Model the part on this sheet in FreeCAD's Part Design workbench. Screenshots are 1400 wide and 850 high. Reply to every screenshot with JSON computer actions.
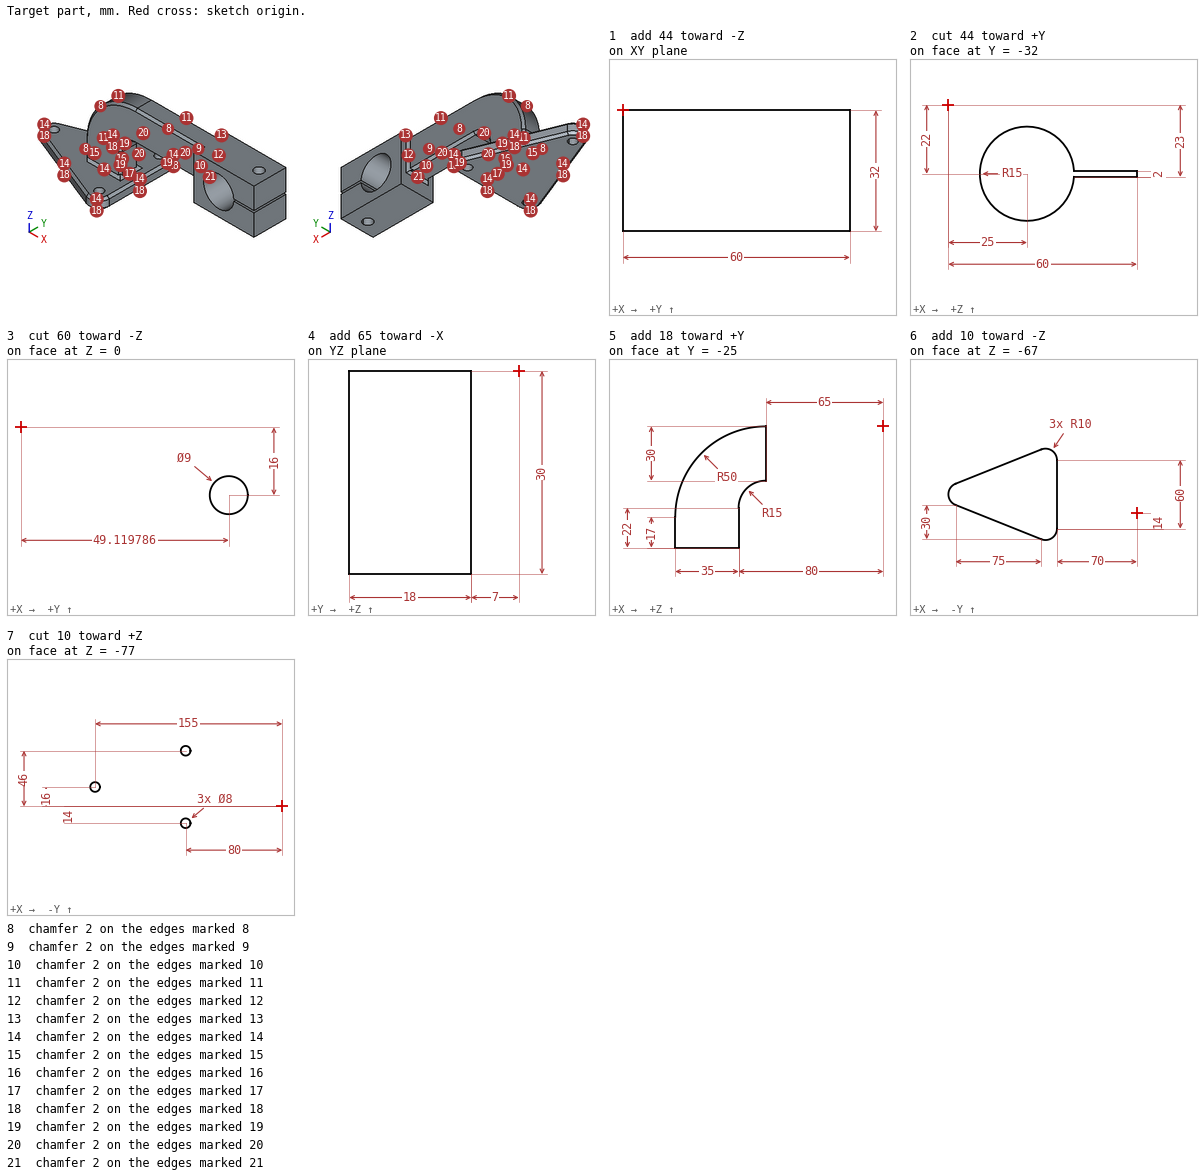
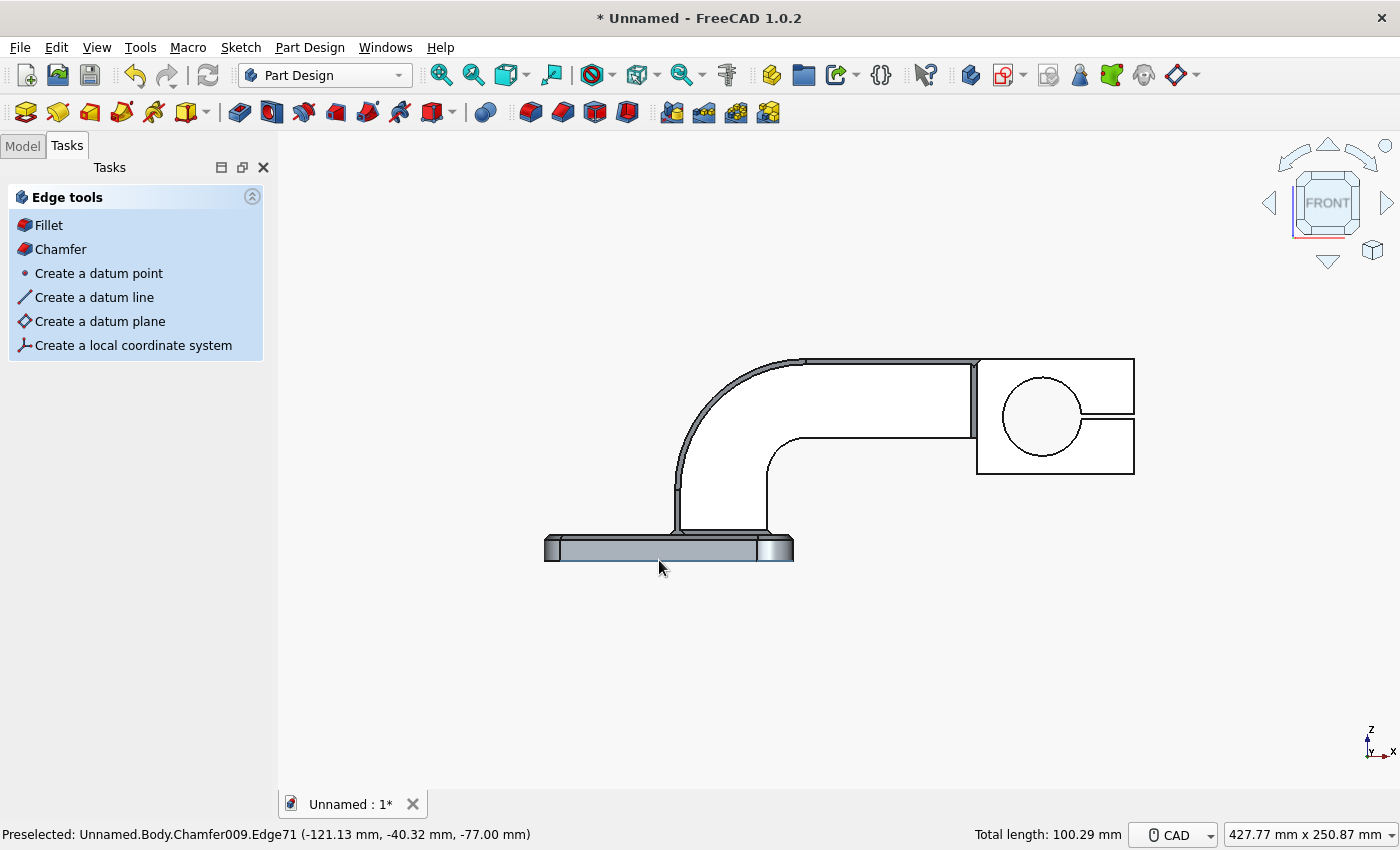
{"action": "left_click", "coordinate": [544, 560], "text": "ctrl"}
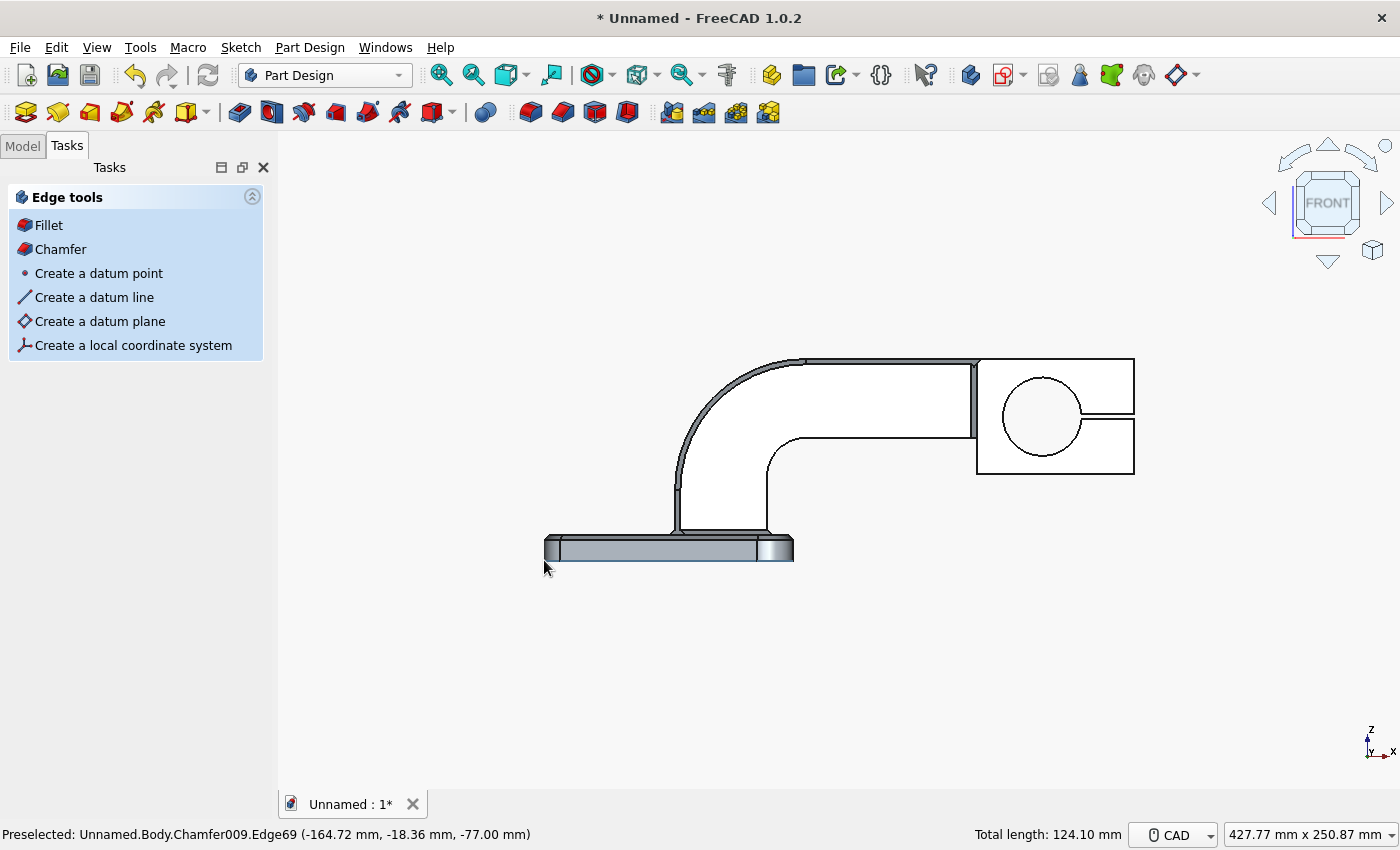
{"action": "key", "text": "3"}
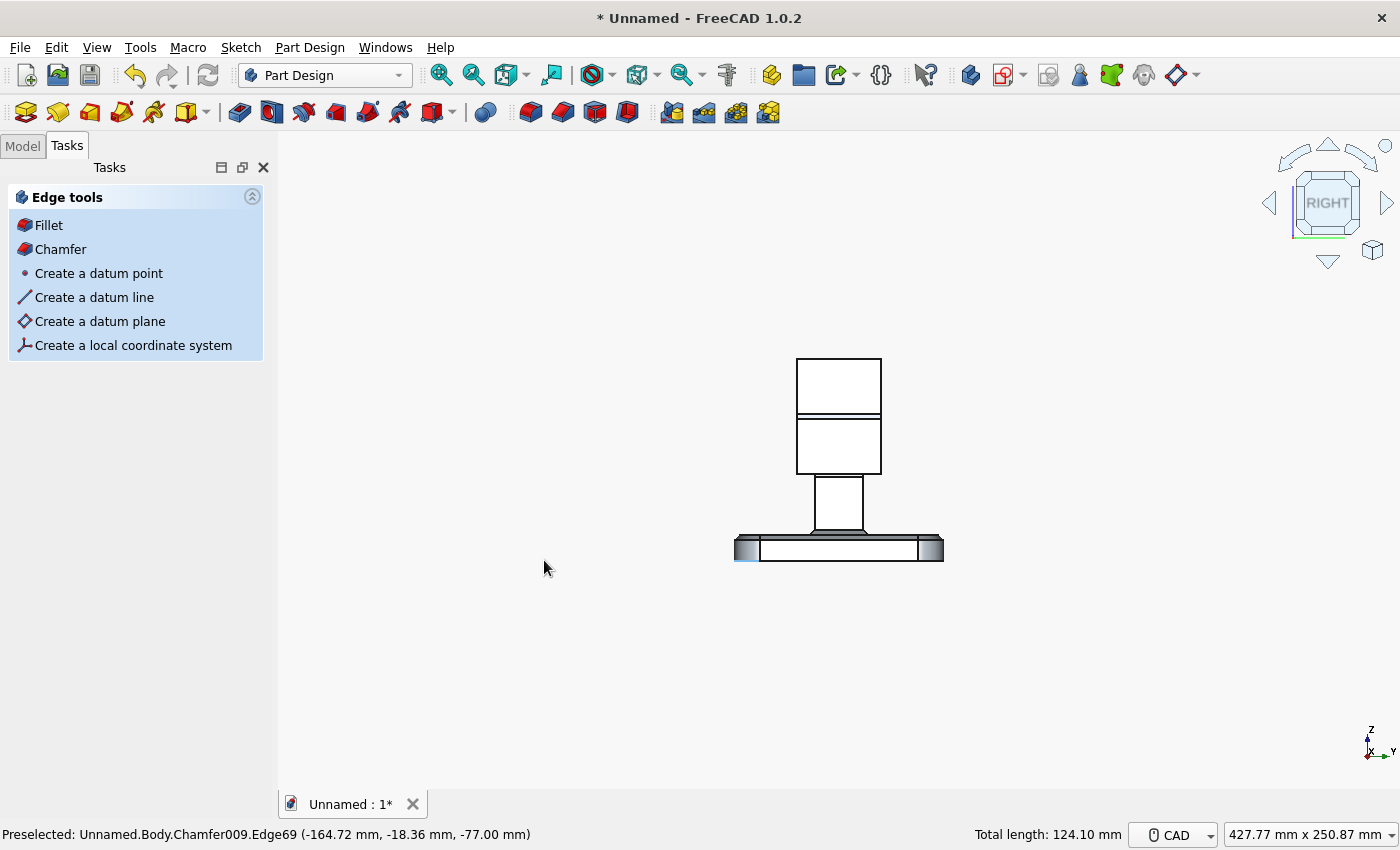
{"action": "left_click", "coordinate": [442, 76]}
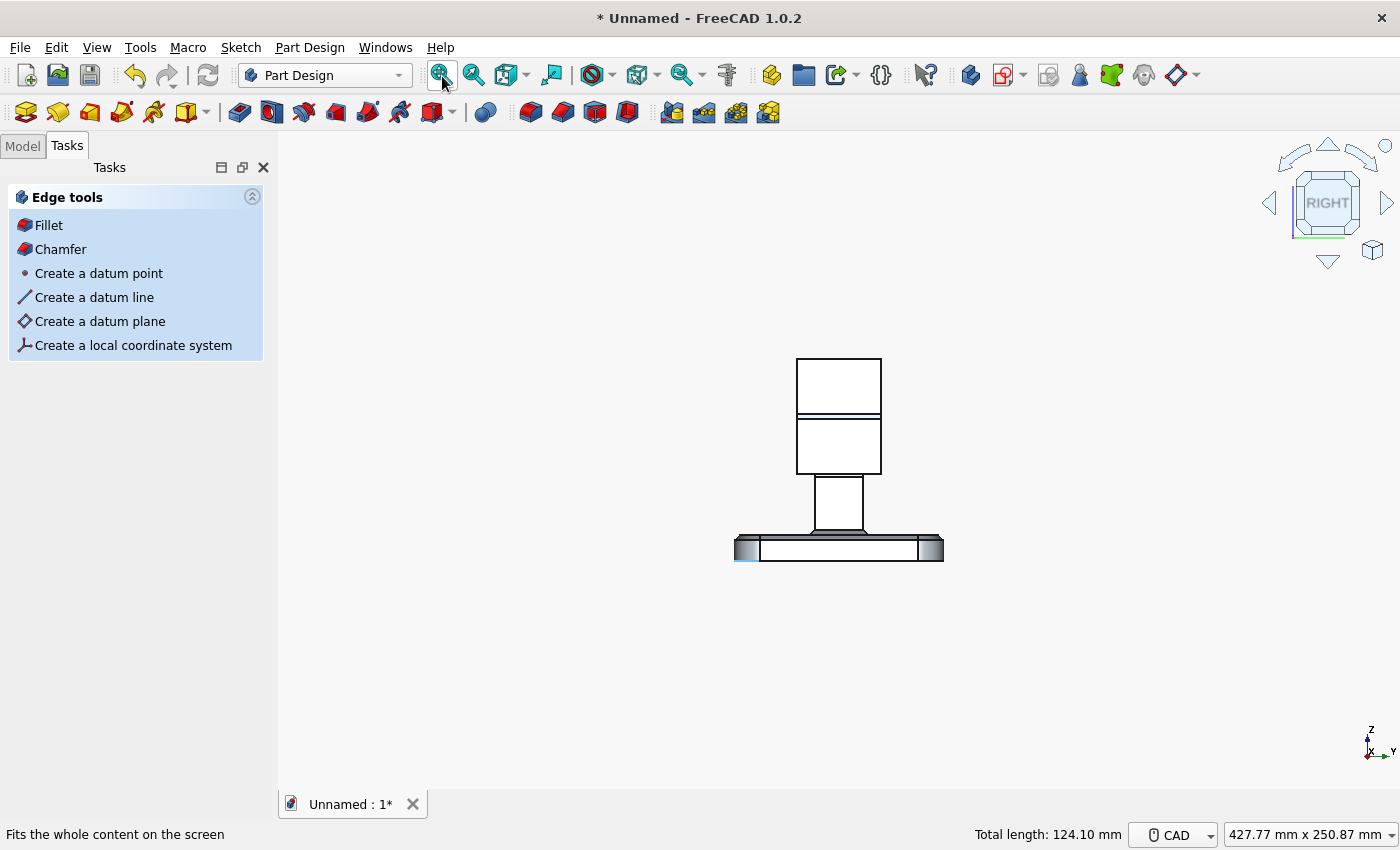
{"action": "left_click", "coordinate": [939, 560], "text": "ctrl"}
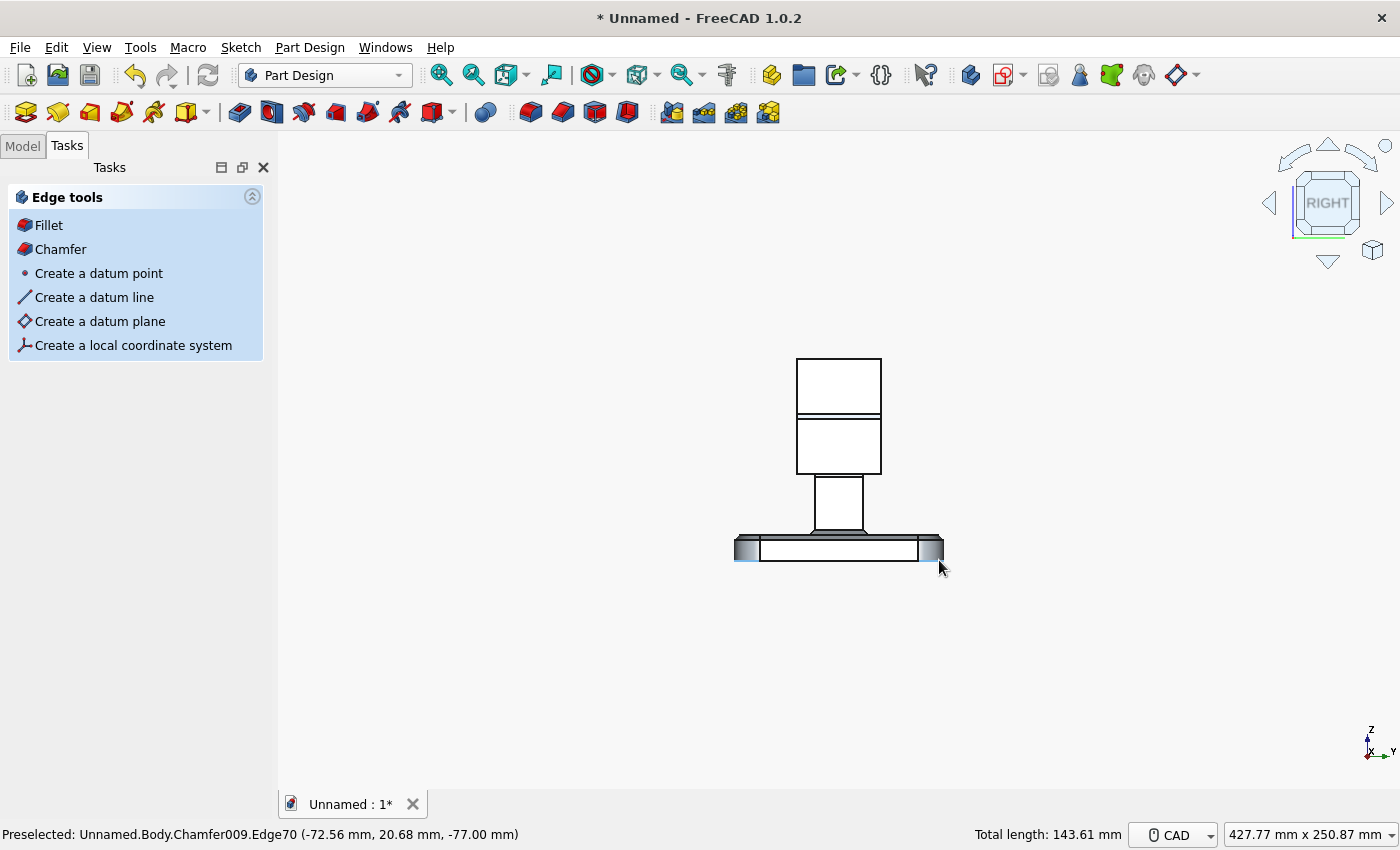
{"action": "left_click", "coordinate": [839, 560], "text": "ctrl"}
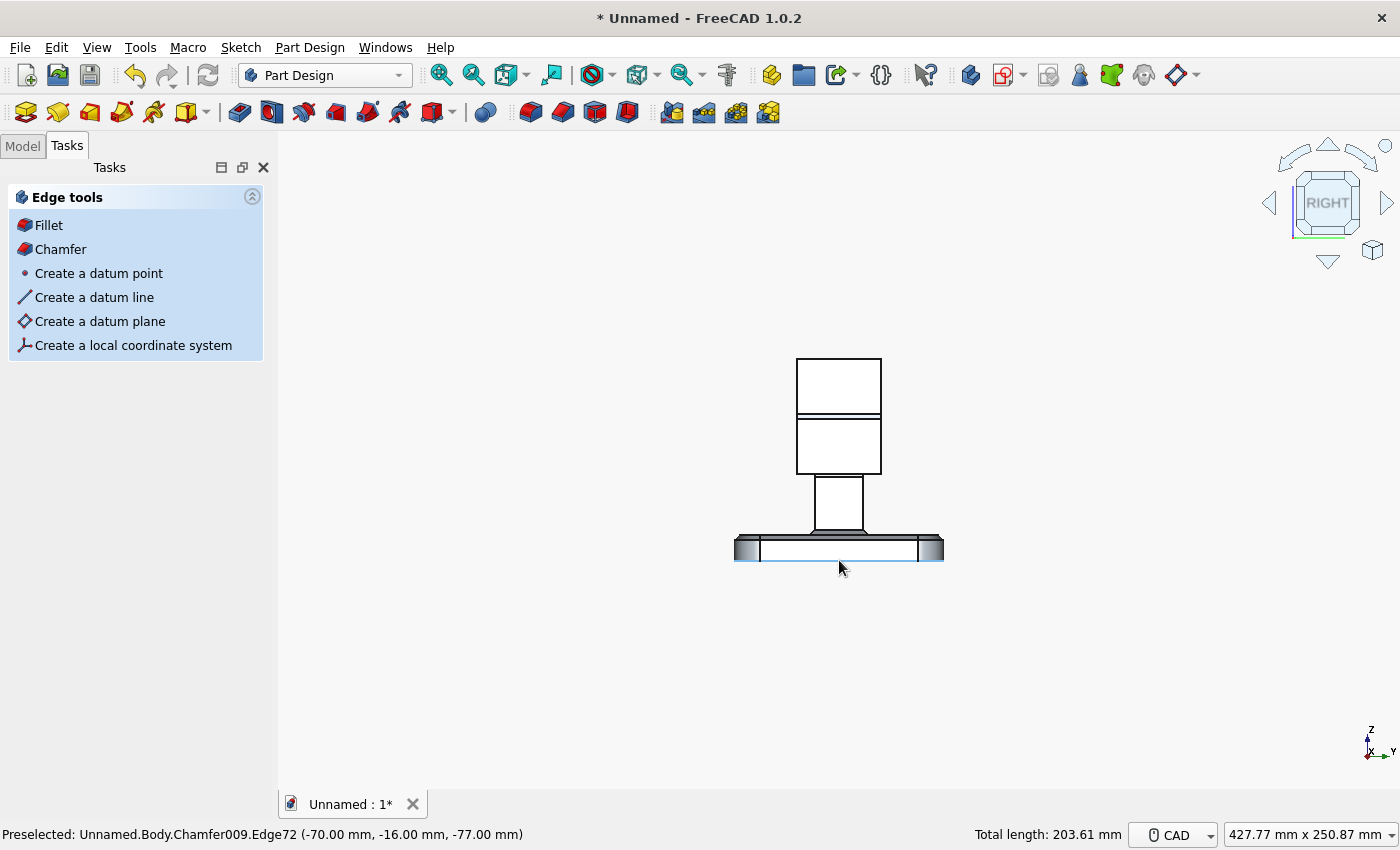
{"action": "key", "text": "5"}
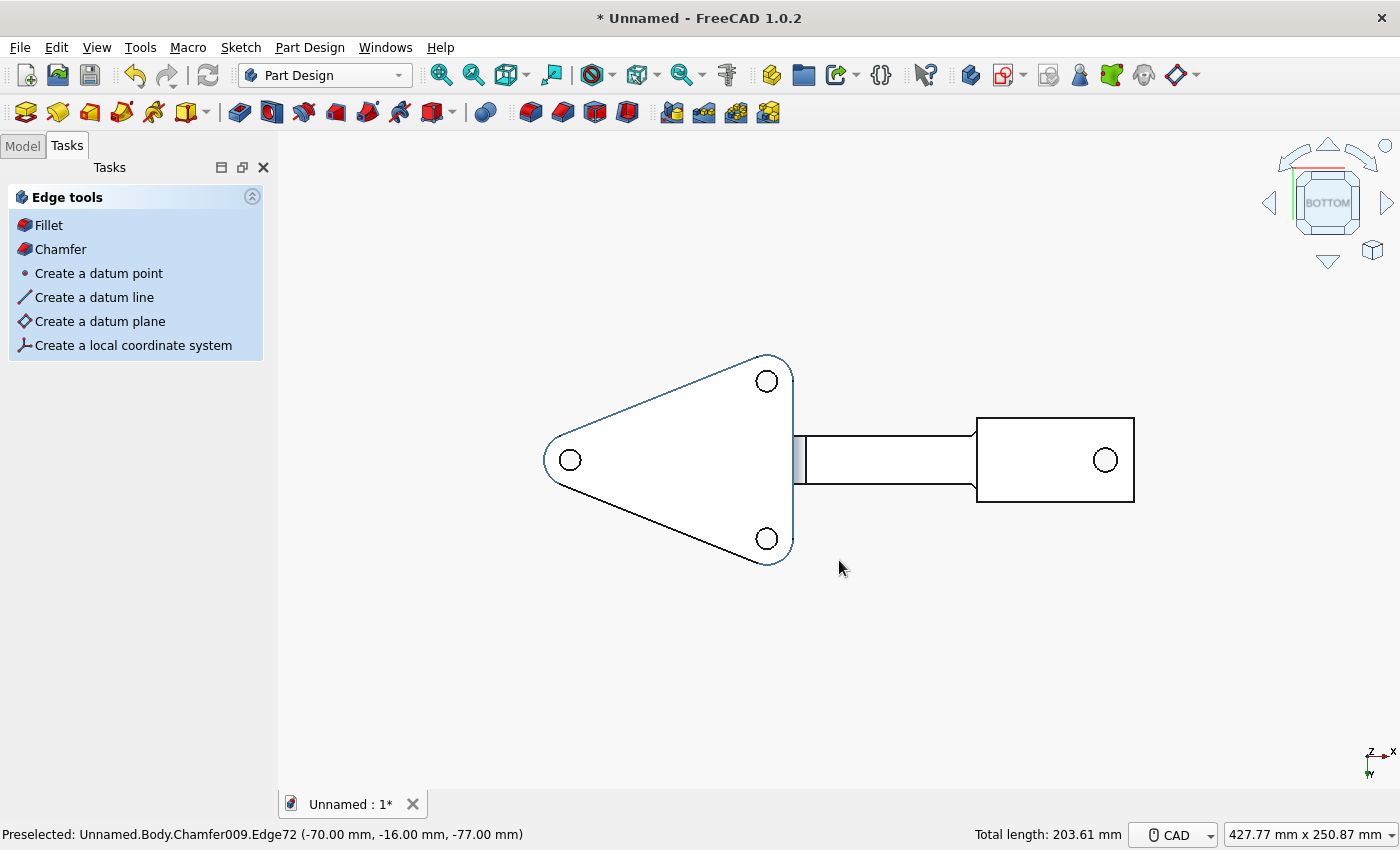
{"action": "left_click", "coordinate": [659, 523], "text": "ctrl"}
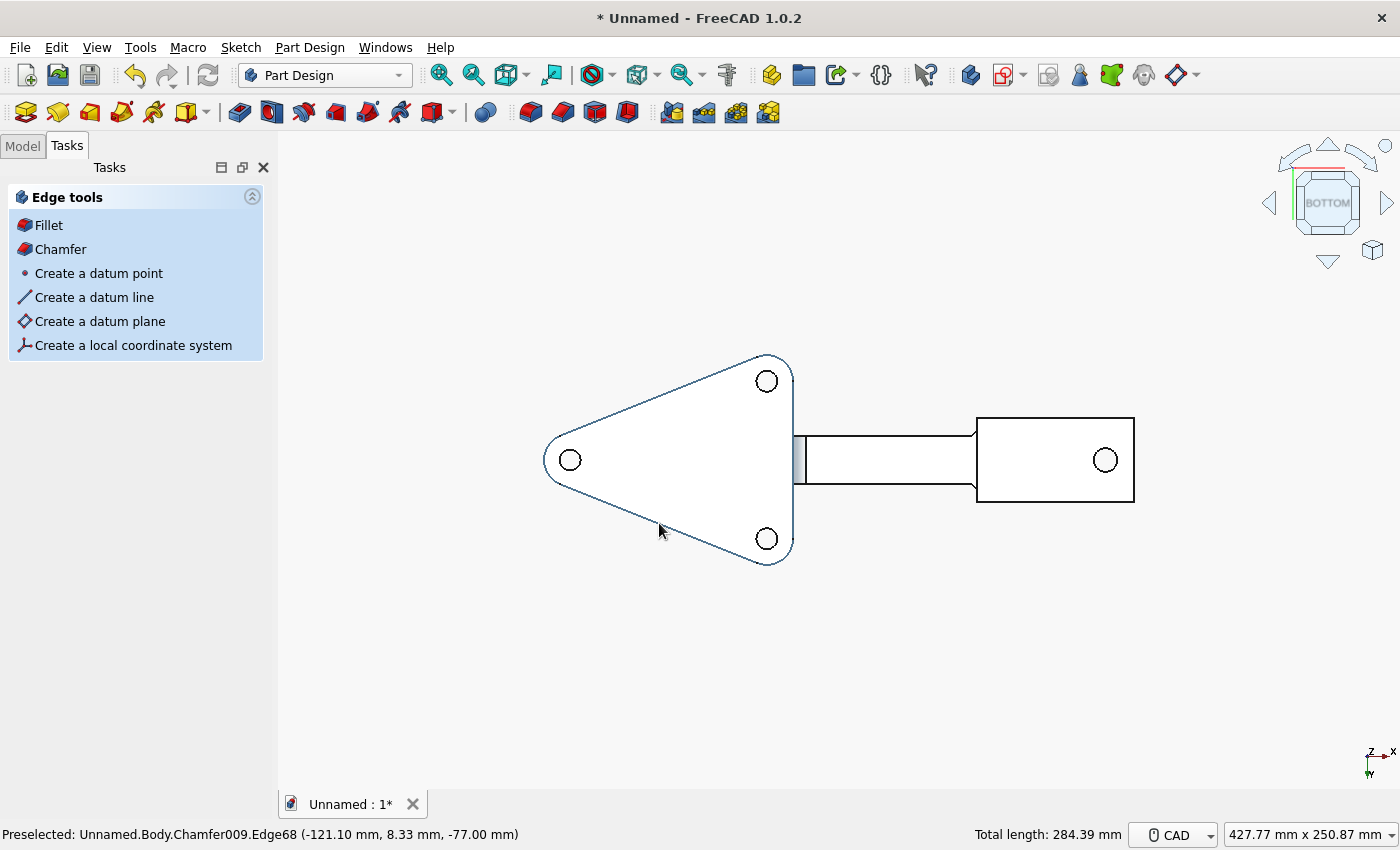
{"action": "left_click", "coordinate": [564, 112]}